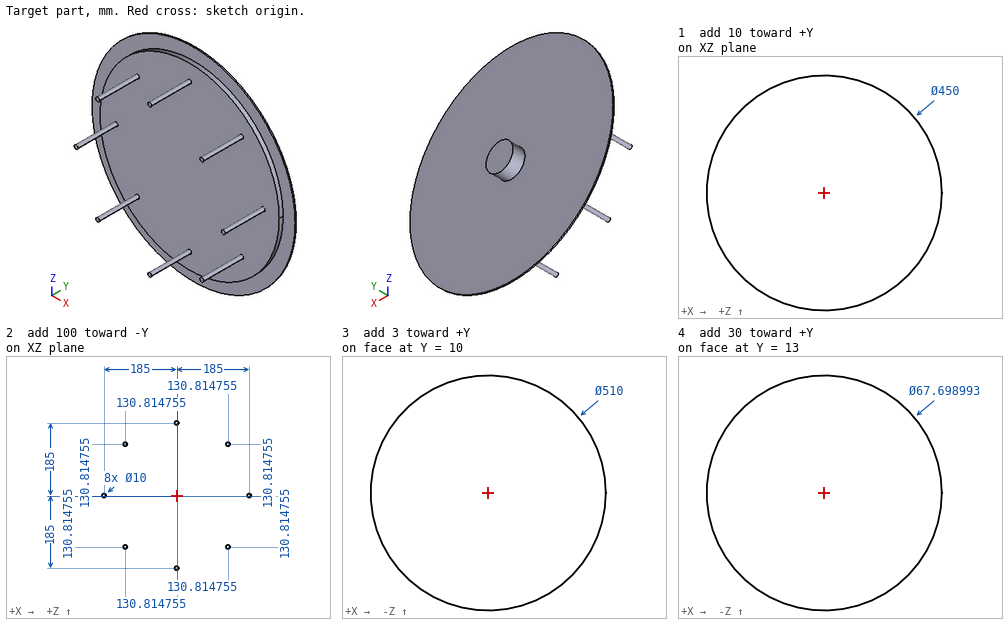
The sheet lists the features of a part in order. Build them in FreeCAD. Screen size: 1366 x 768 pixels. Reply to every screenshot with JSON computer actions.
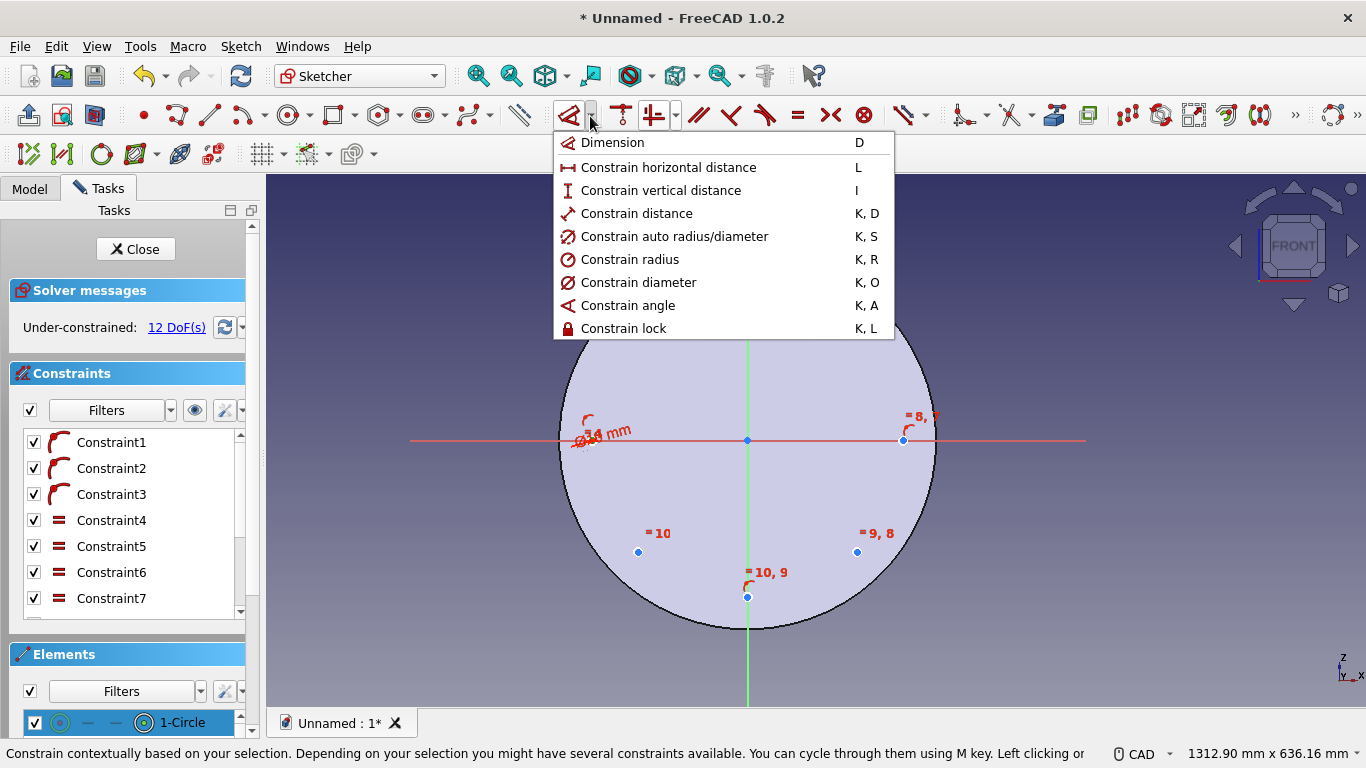
{"action": "left_click", "coordinate": [724, 168]}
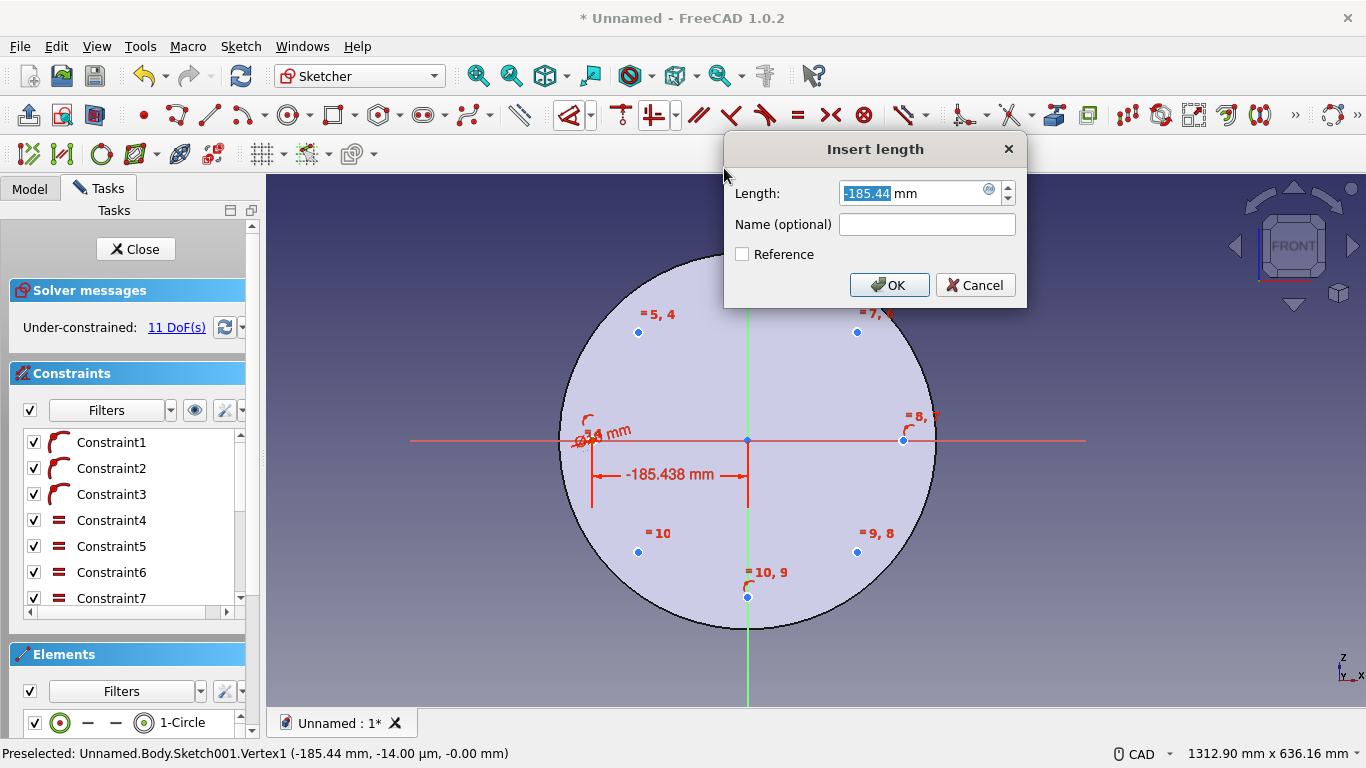
{"action": "type", "text": "-185"}
{"action": "key", "text": "Return"}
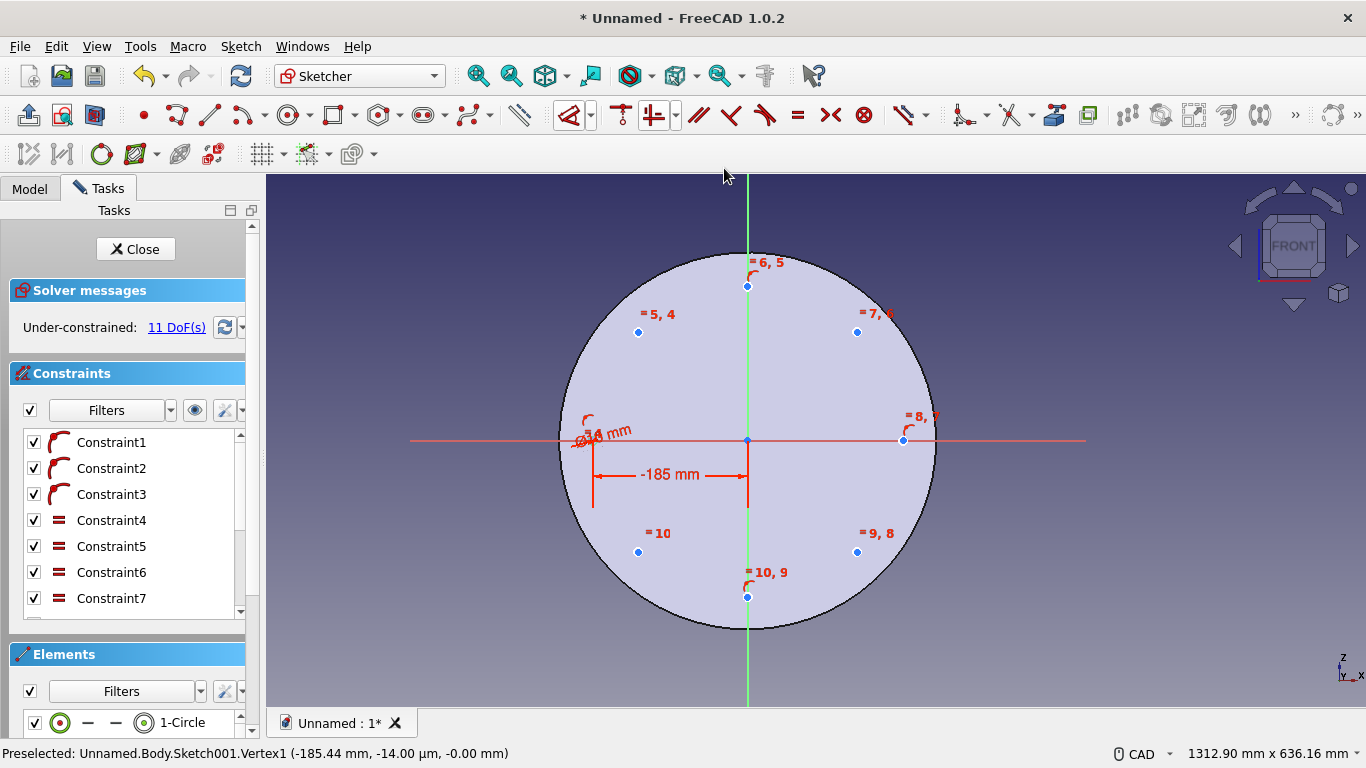
{"action": "left_click", "coordinate": [748, 287]}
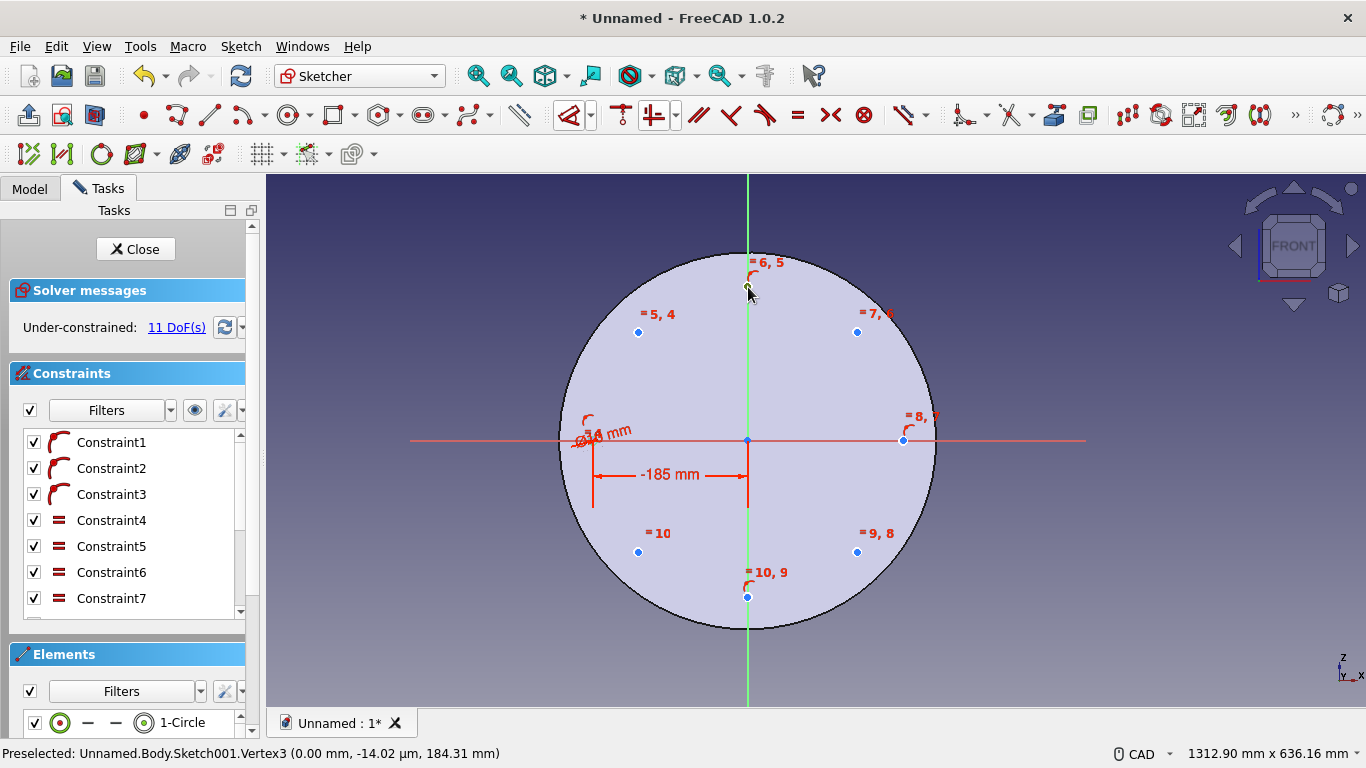
{"action": "left_click", "coordinate": [590, 116]}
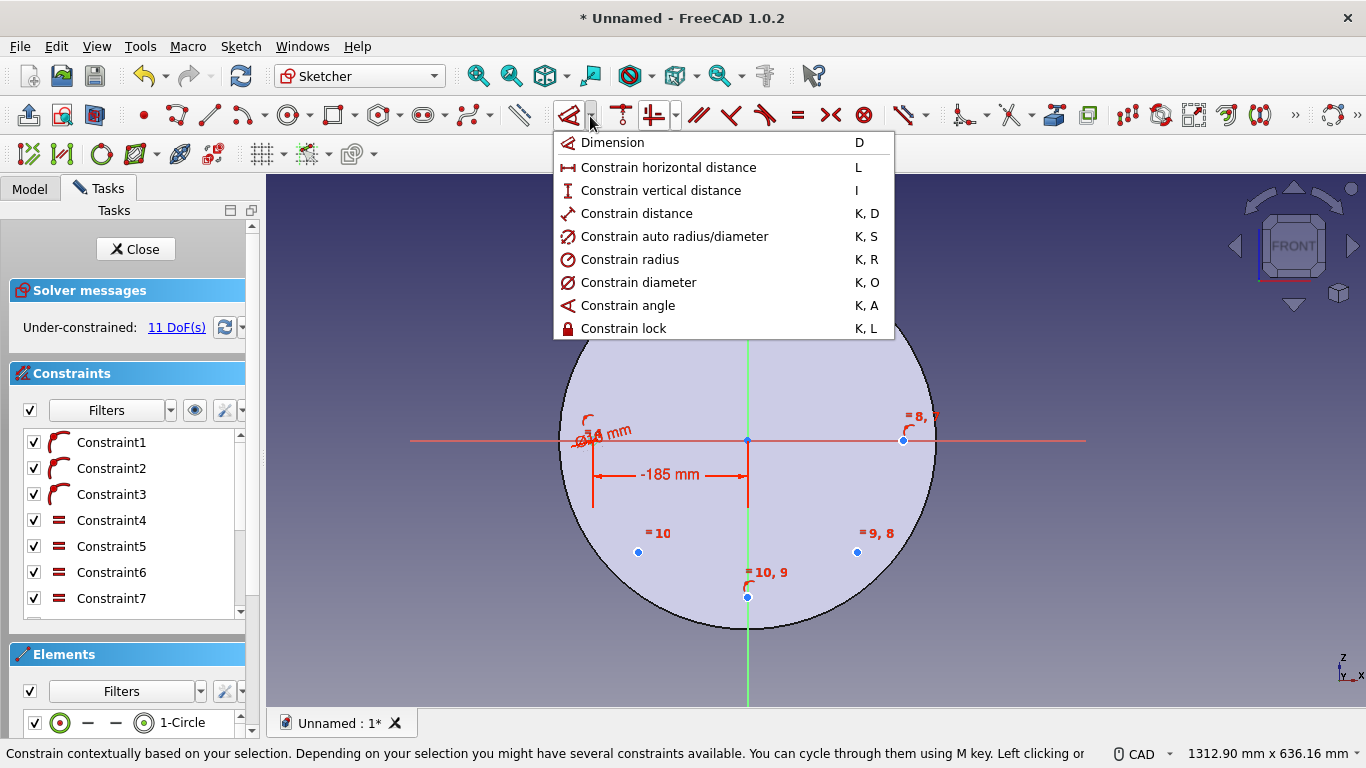
{"action": "left_click", "coordinate": [724, 190]}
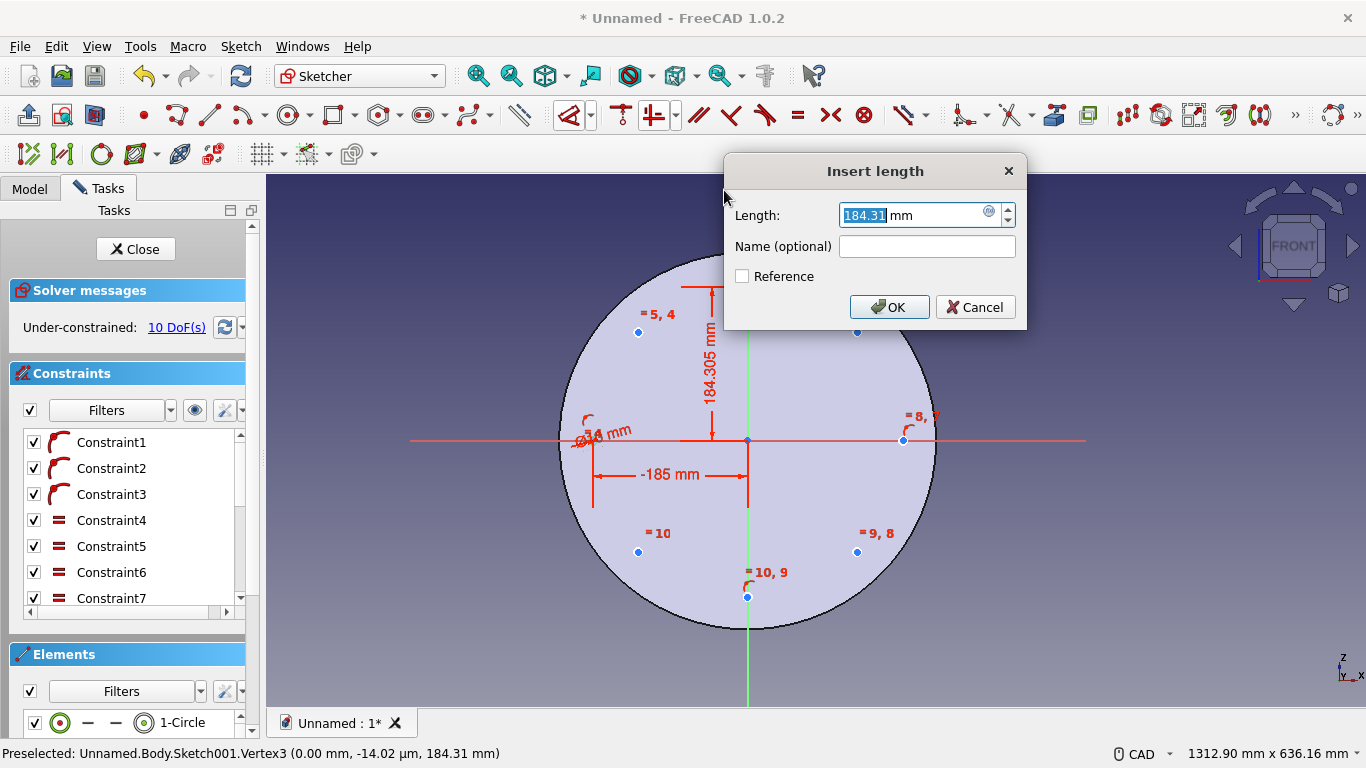
{"action": "type", "text": "185"}
{"action": "key", "text": "Return"}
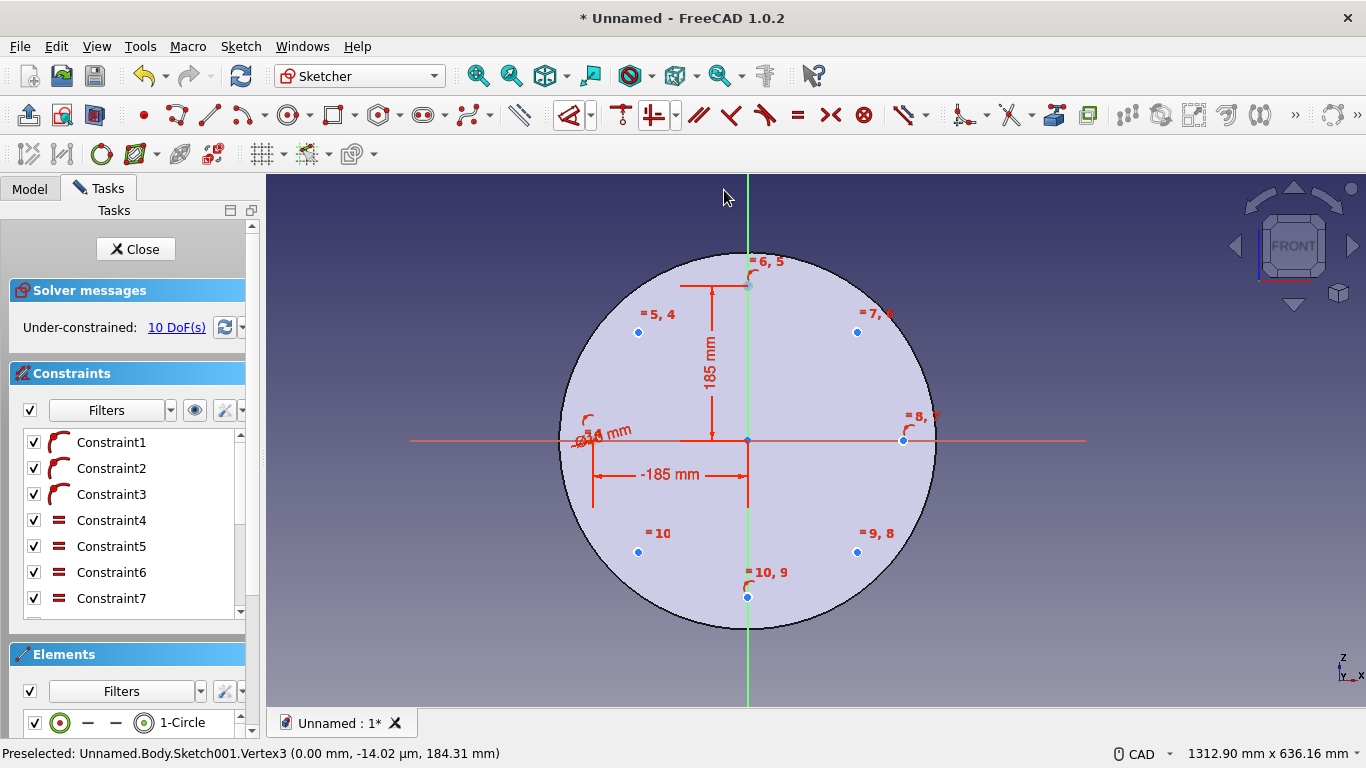
{"action": "left_click", "coordinate": [903, 441]}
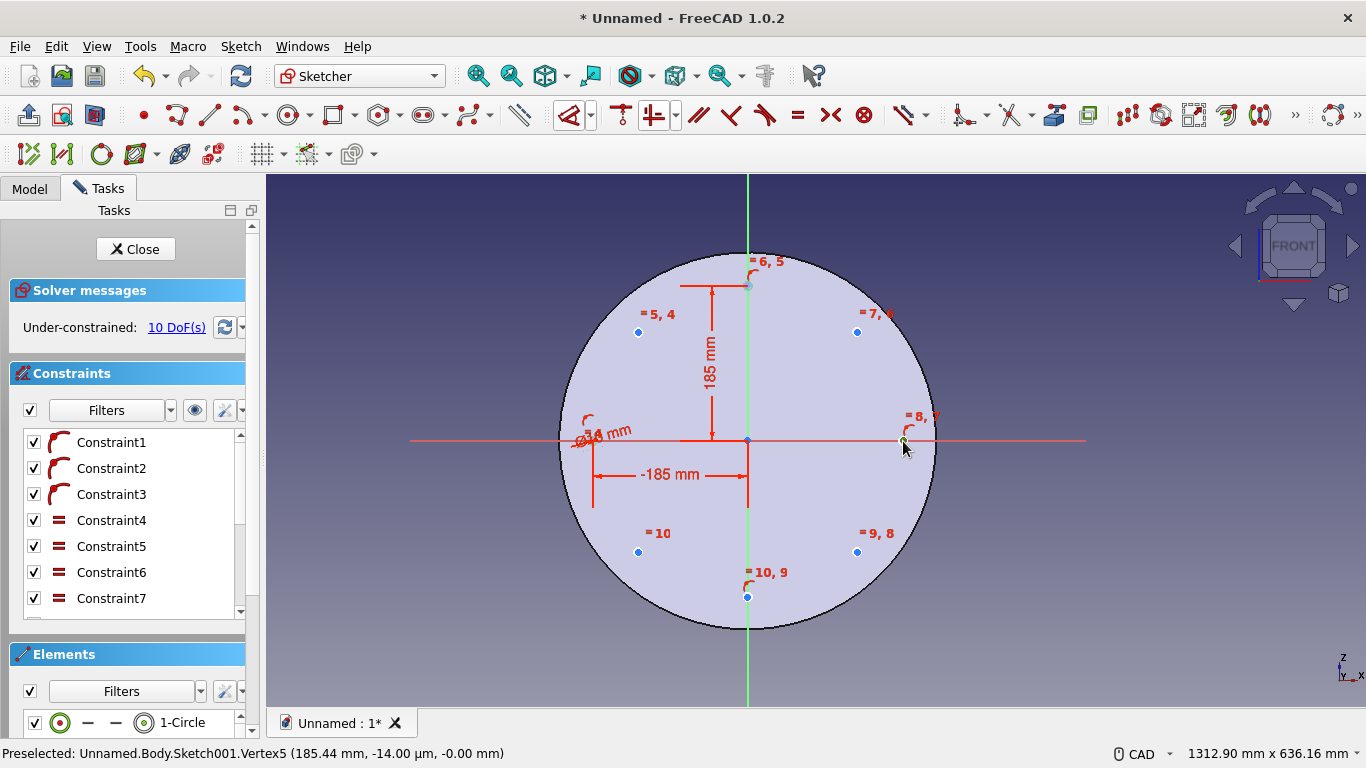
{"action": "key", "text": "l"}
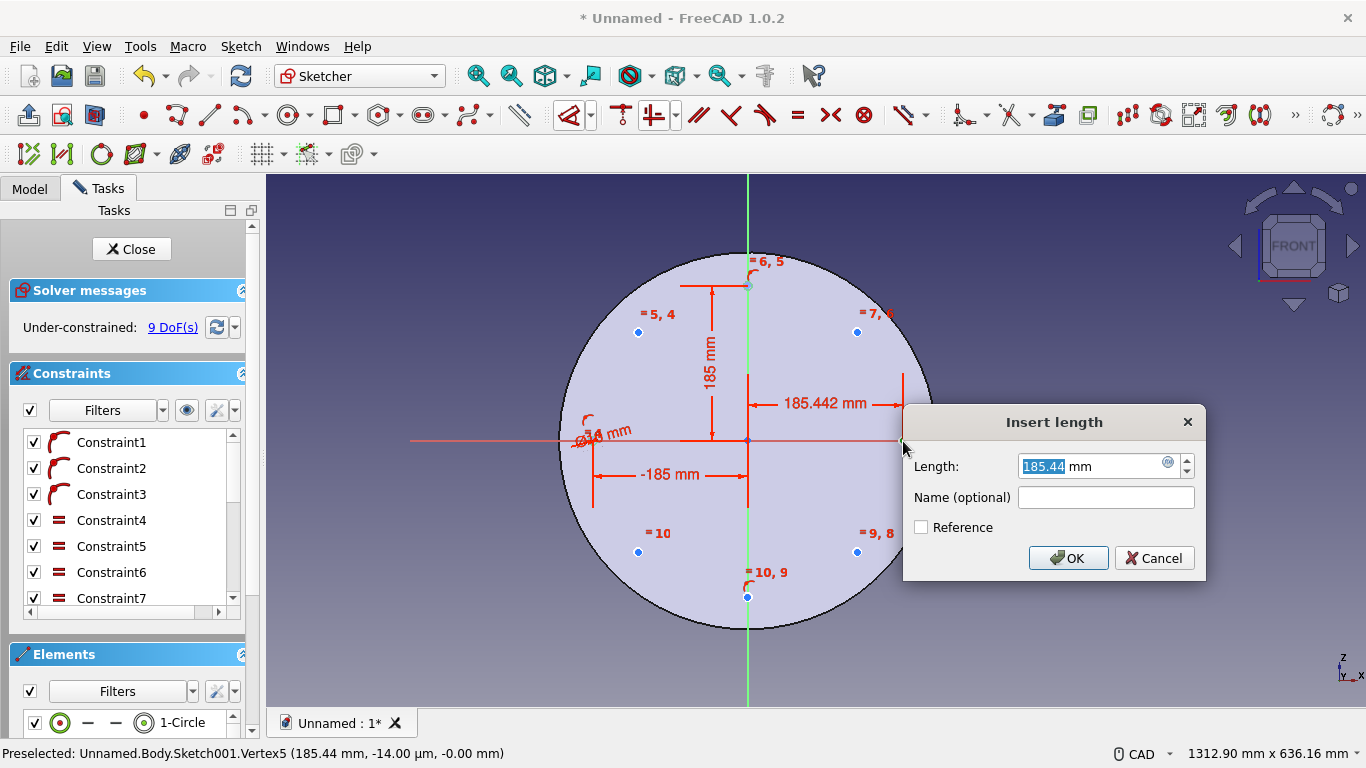
{"action": "type", "text": "185"}
{"action": "key", "text": "Return"}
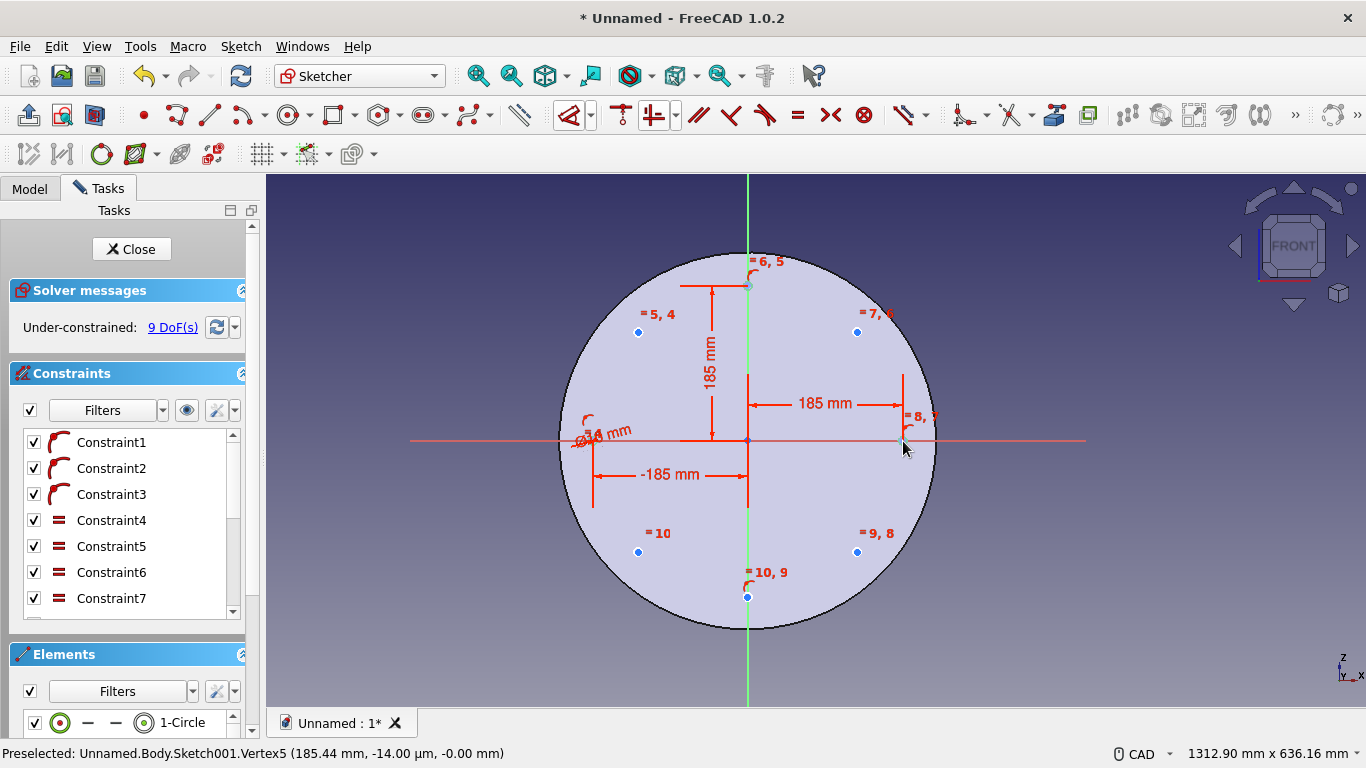
{"action": "left_click", "coordinate": [748, 597]}